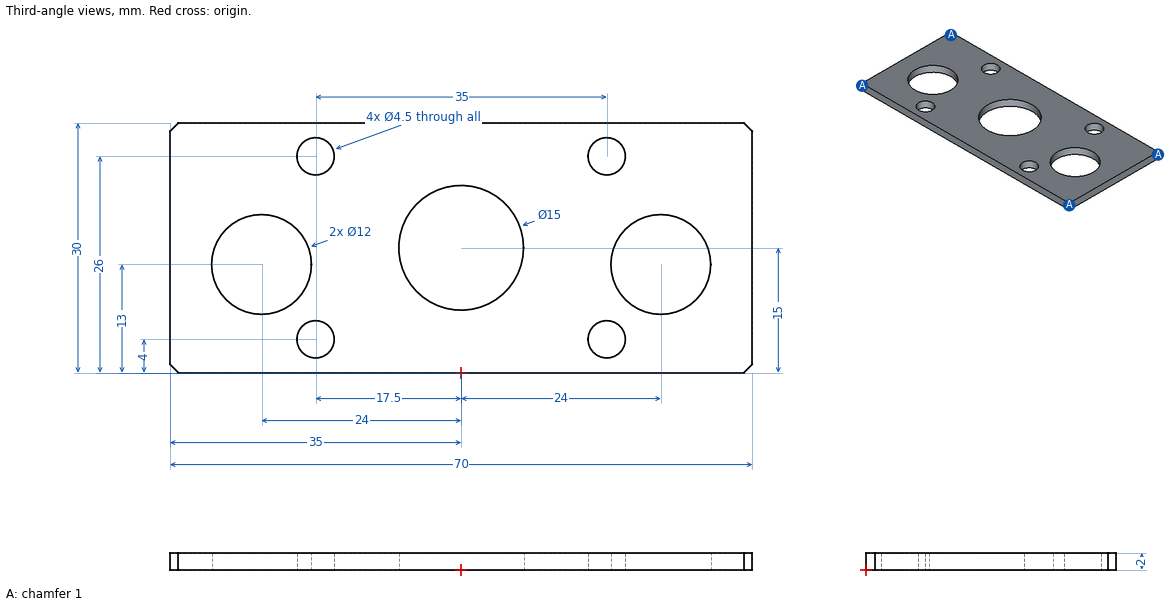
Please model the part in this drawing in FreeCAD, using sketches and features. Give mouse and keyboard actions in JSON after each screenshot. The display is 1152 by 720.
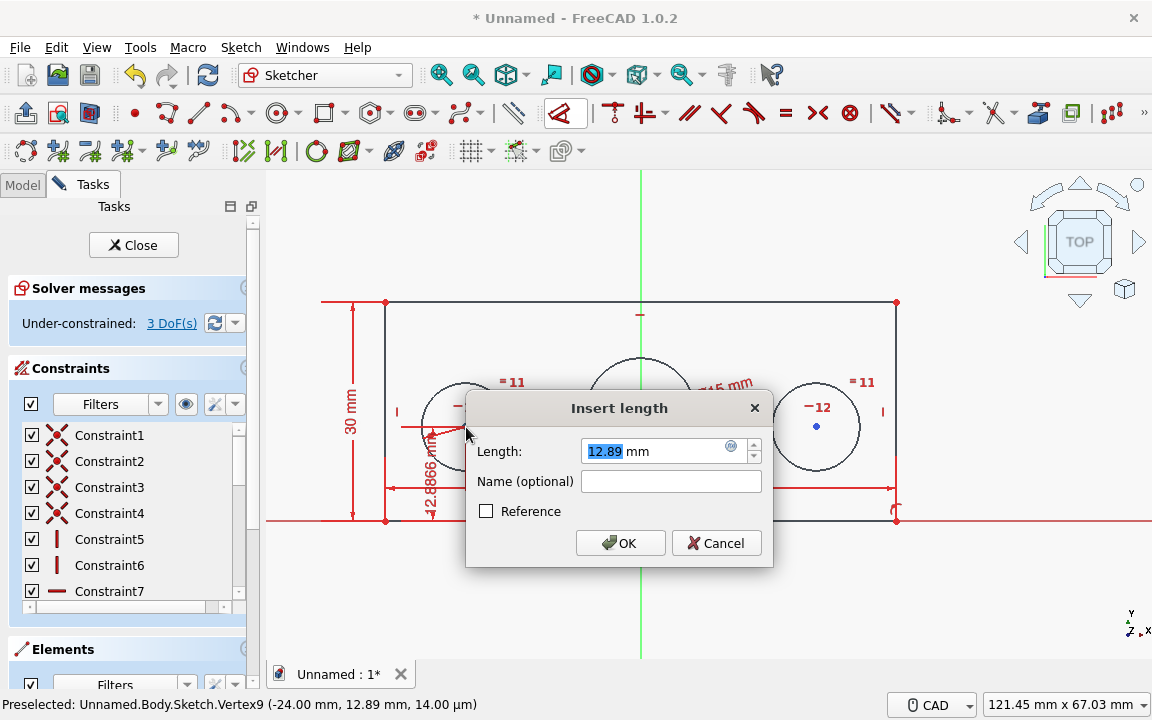
{"action": "type", "text": "13"}
{"action": "key", "text": "Return"}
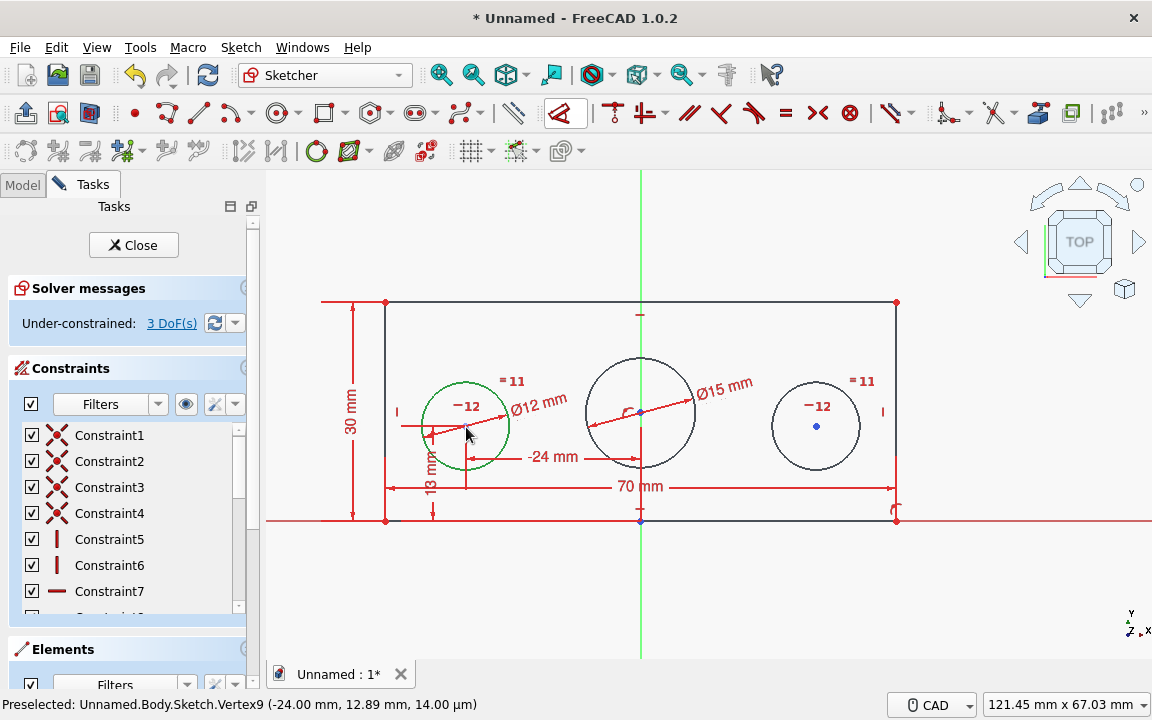
{"action": "left_click", "coordinate": [816, 426]}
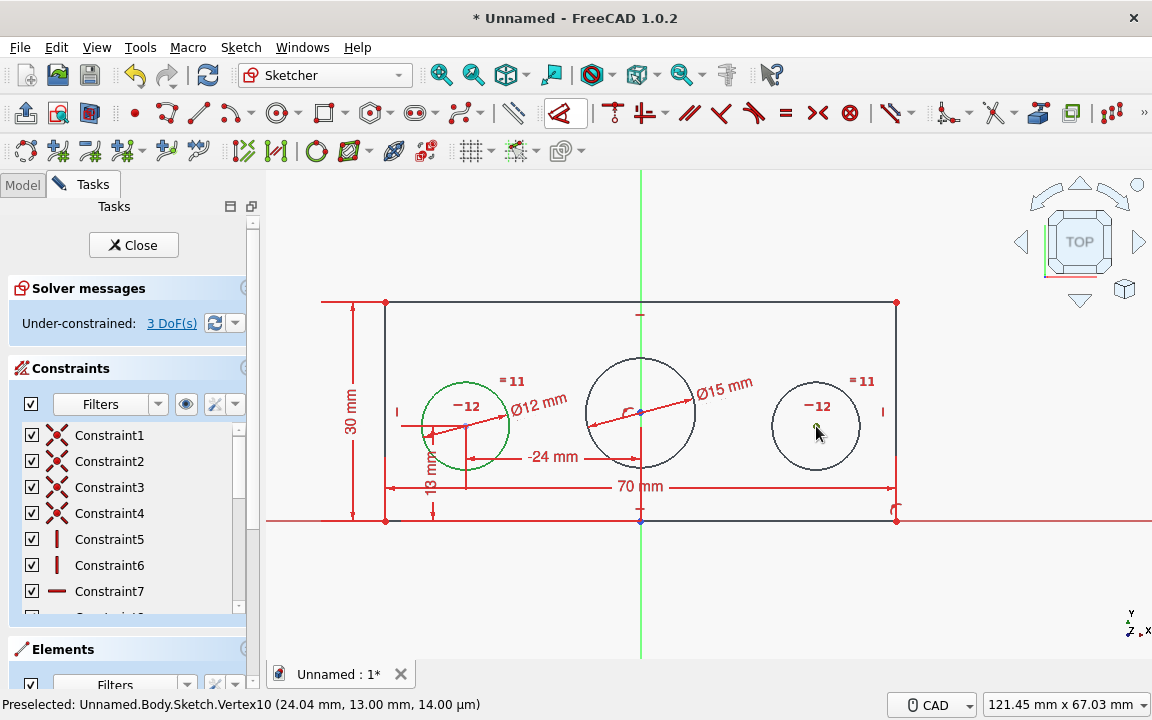
{"action": "left_click", "coordinate": [582, 114]}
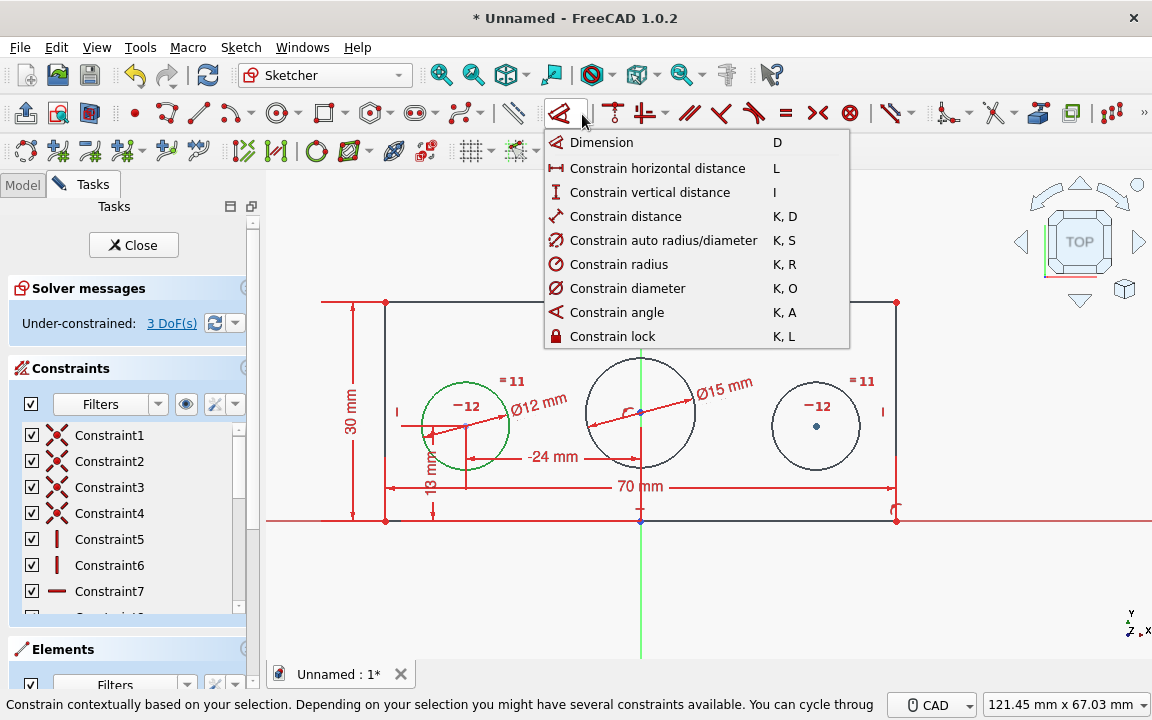
{"action": "left_click", "coordinate": [697, 168]}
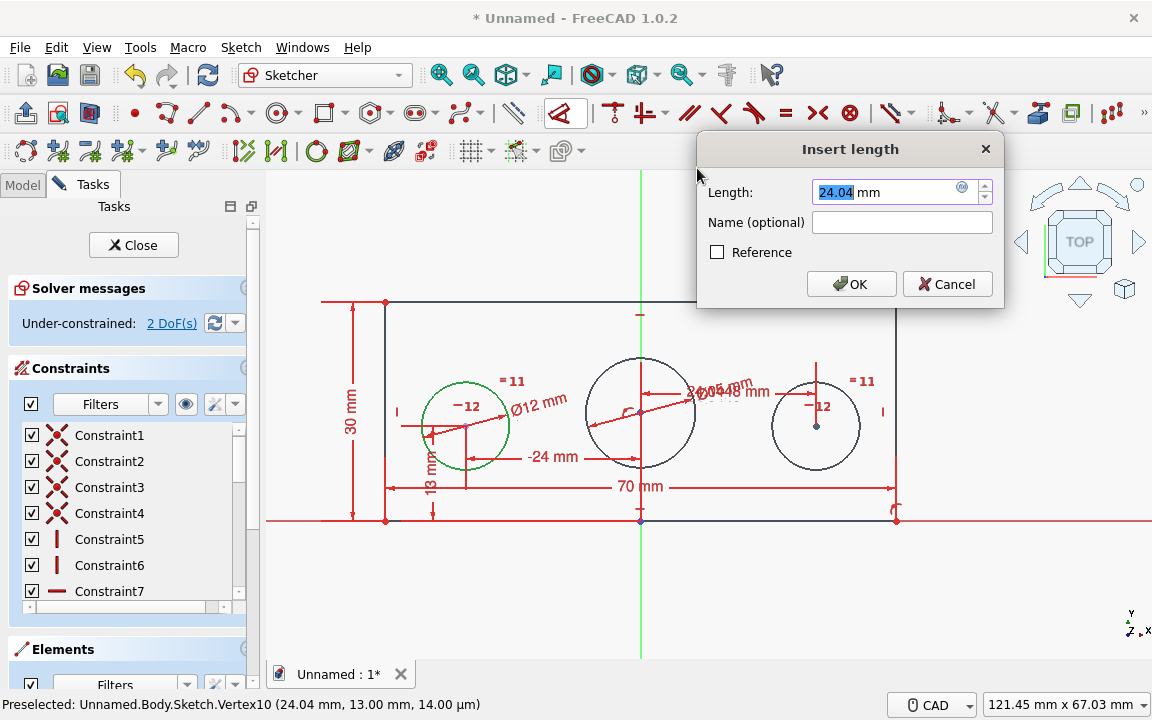
{"action": "type", "text": "24"}
{"action": "key", "text": "Return"}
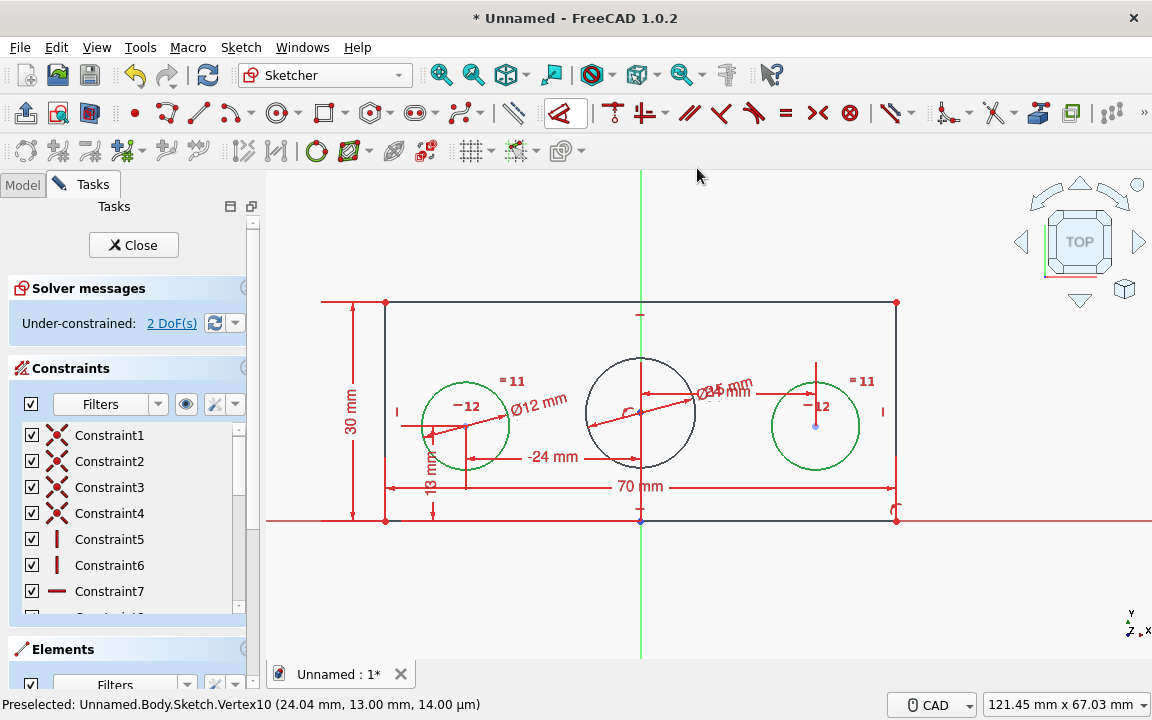
{"action": "left_click", "coordinate": [641, 413]}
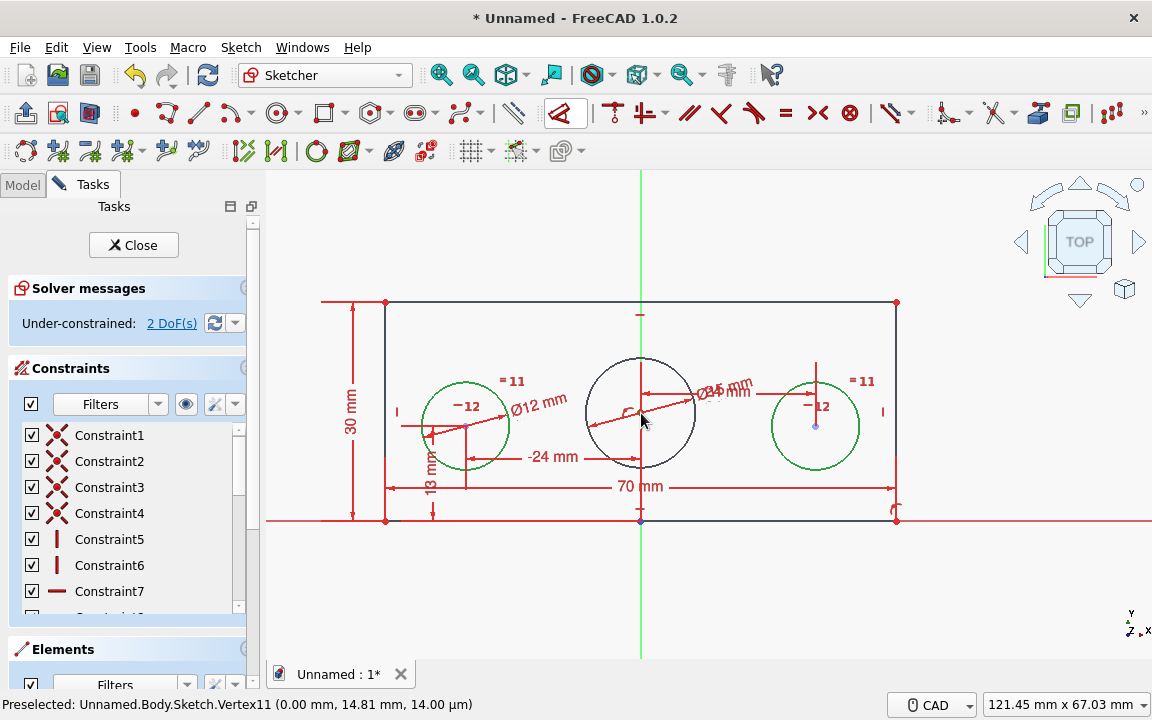
{"action": "key", "text": "i"}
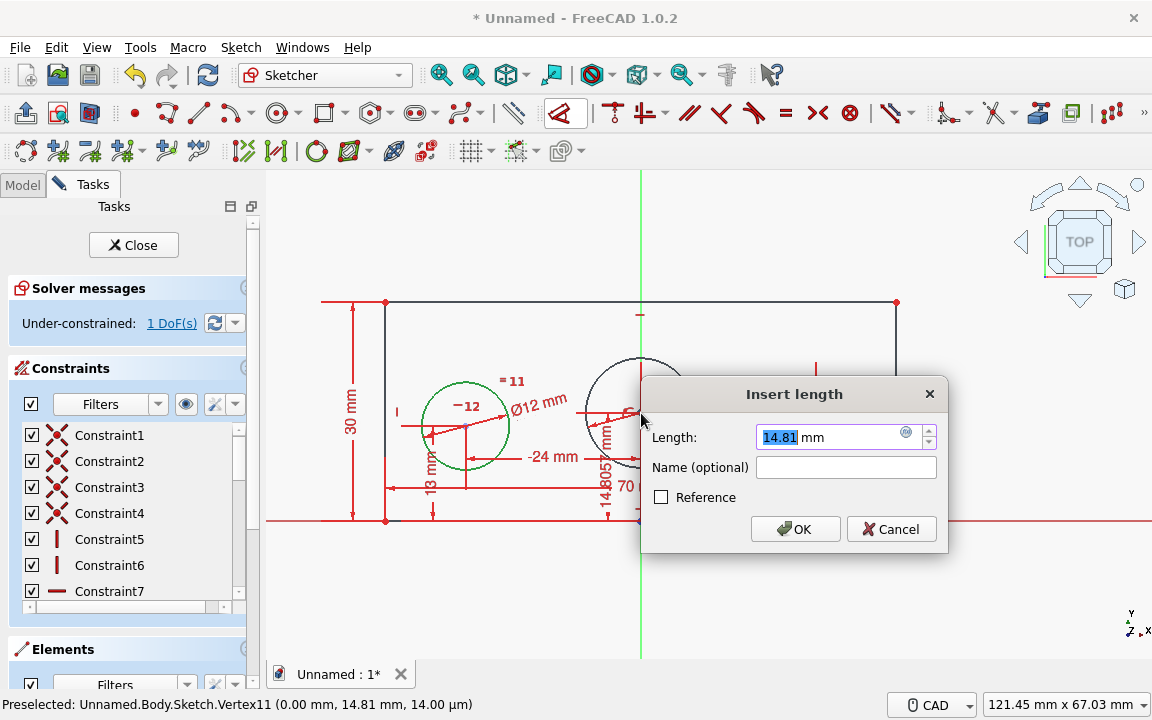
{"action": "type", "text": "15"}
{"action": "key", "text": "Return"}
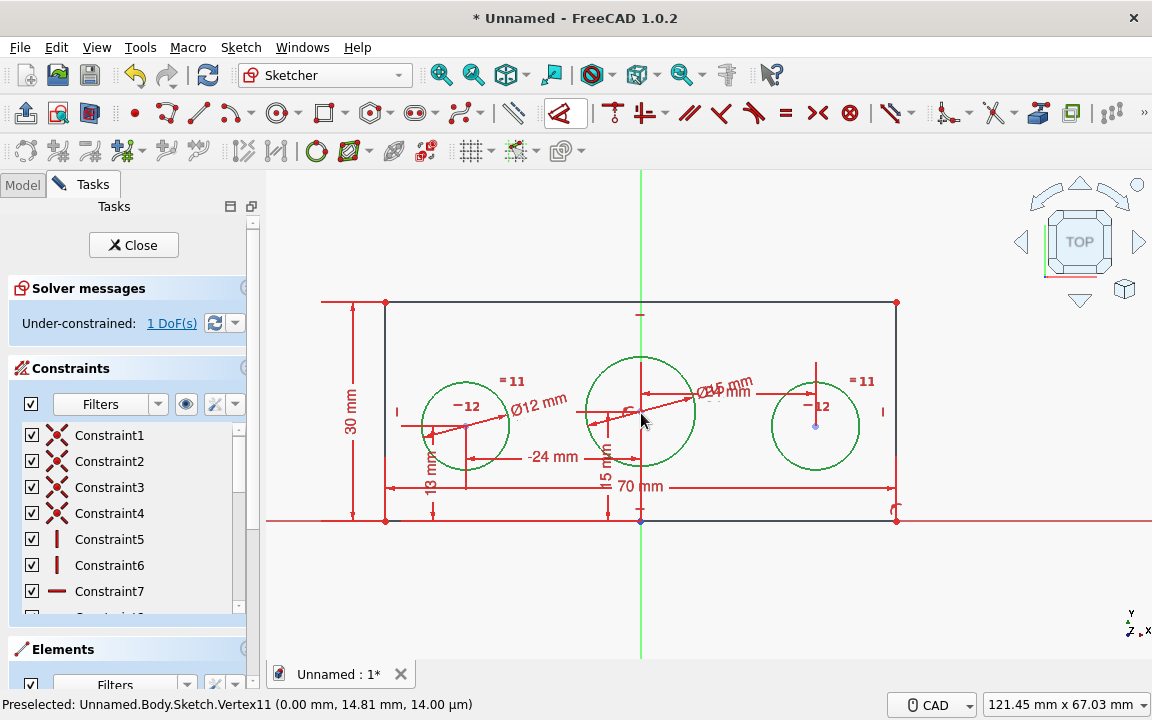
{"action": "left_click", "coordinate": [385, 302]}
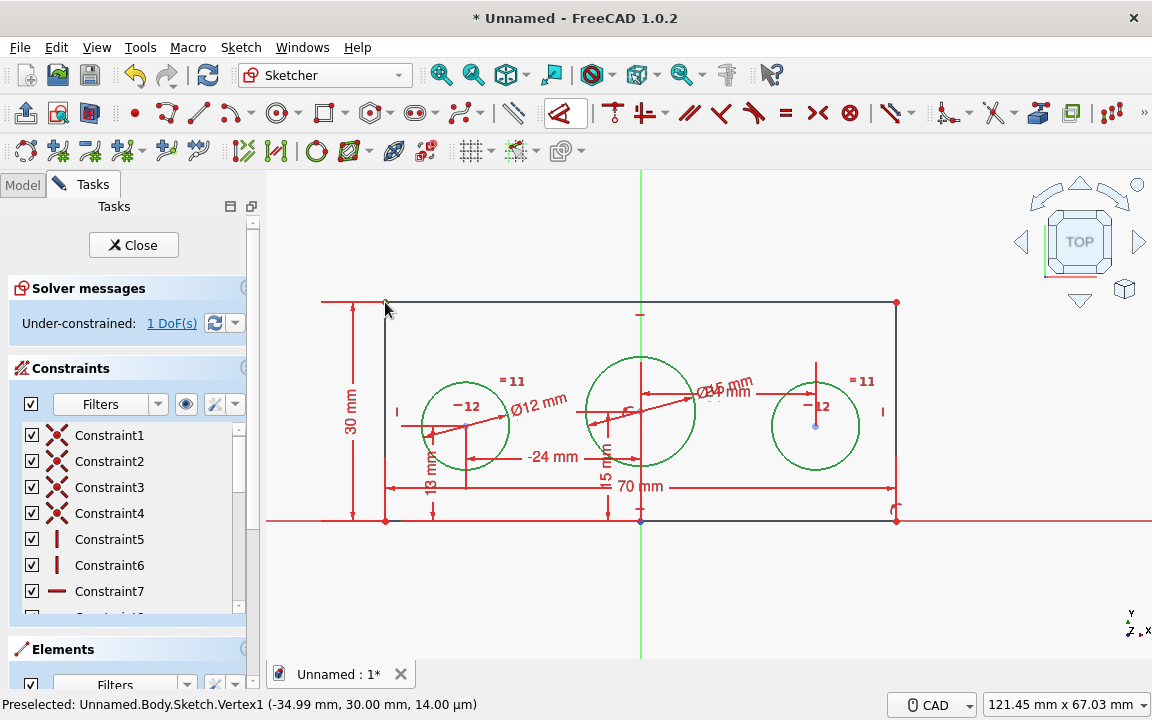
{"action": "key", "text": "l"}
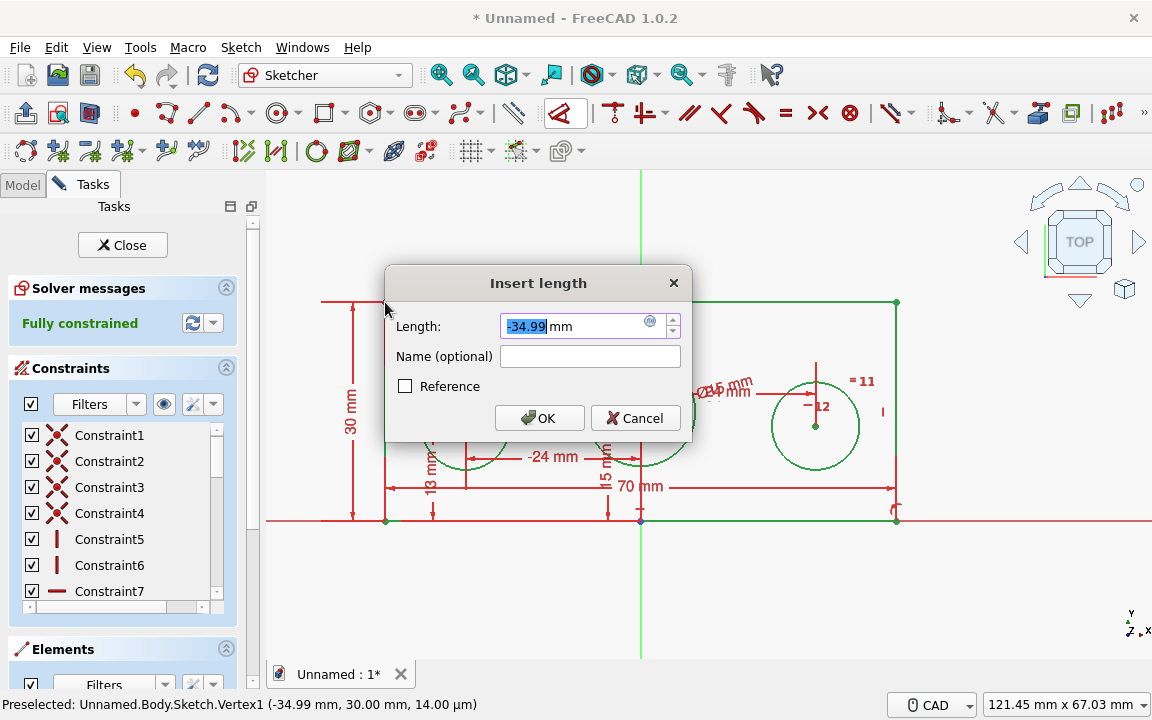
{"action": "type", "text": "-35"}
{"action": "key", "text": "Return"}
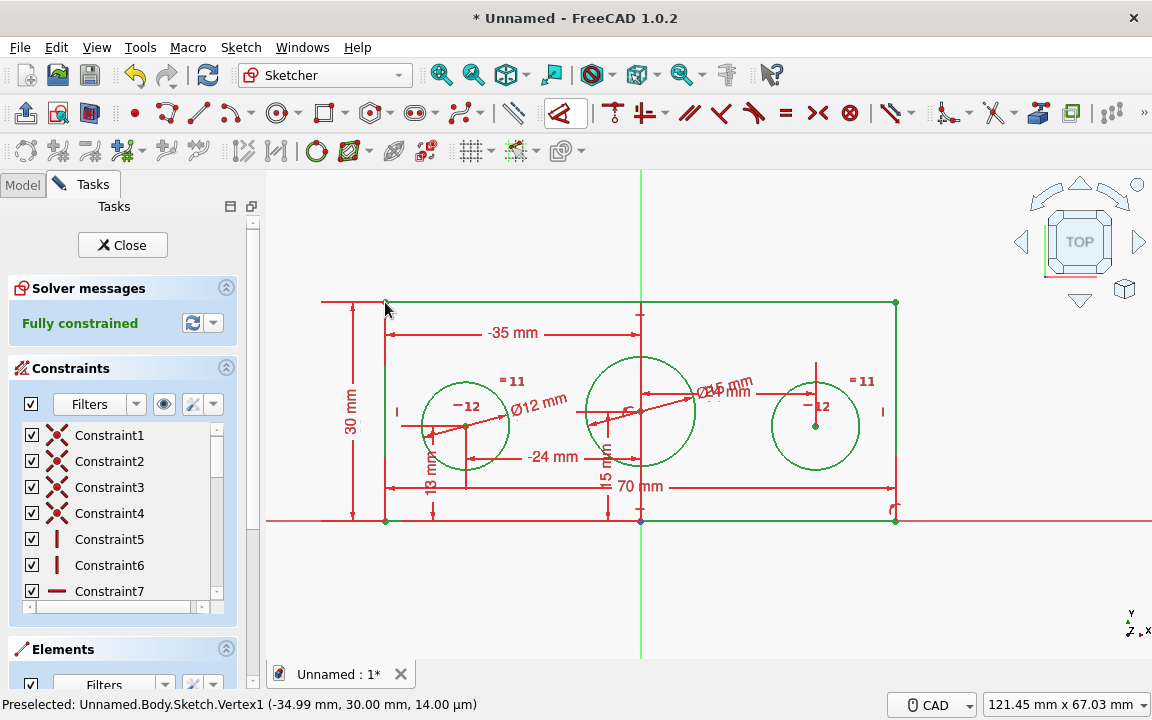
{"action": "left_click", "coordinate": [123, 245]}